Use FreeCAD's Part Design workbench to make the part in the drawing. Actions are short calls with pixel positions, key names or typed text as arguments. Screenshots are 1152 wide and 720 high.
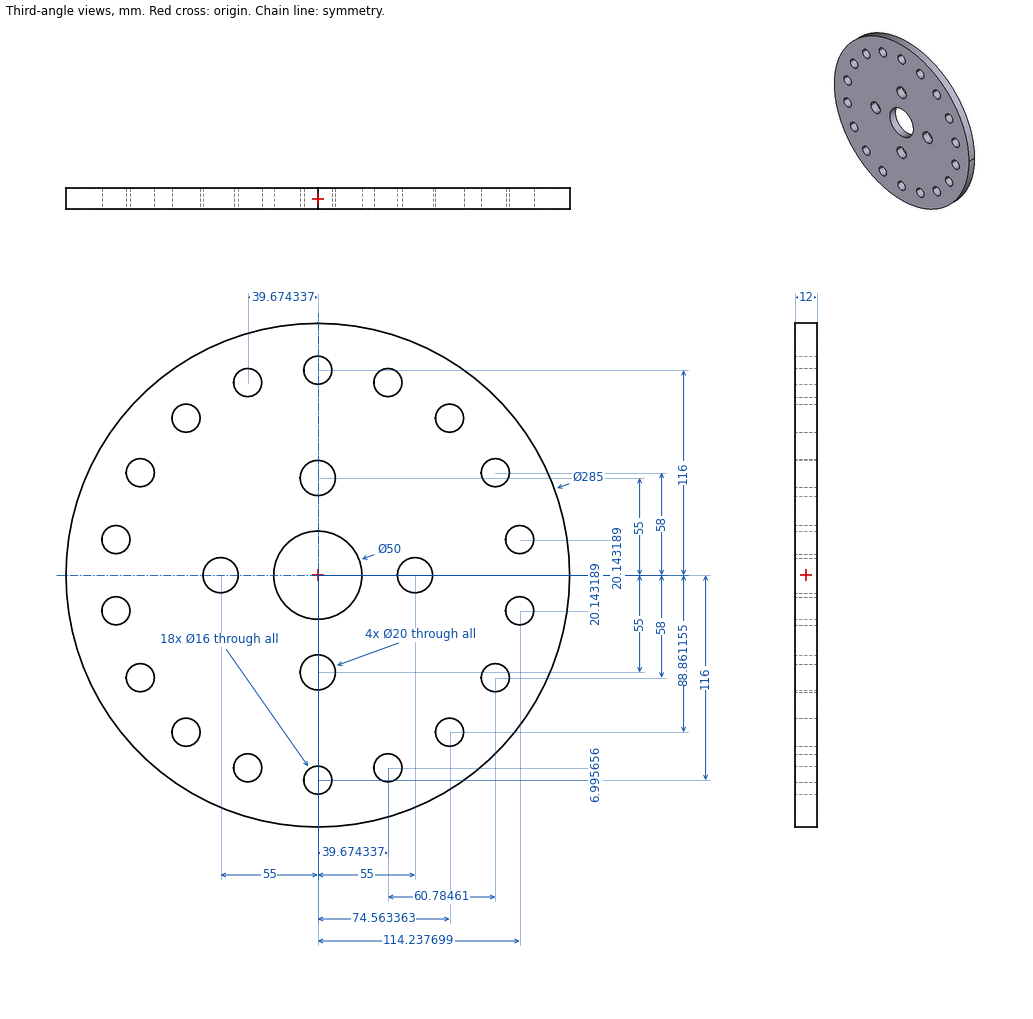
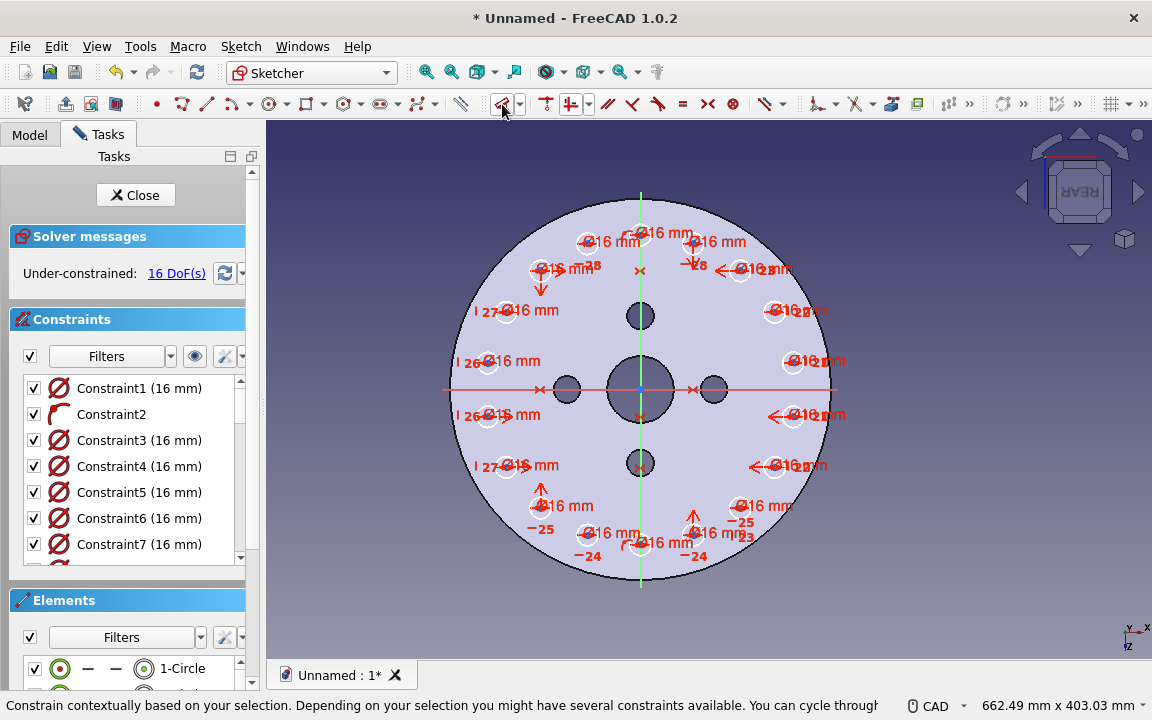
click(775, 312)
click(809, 333)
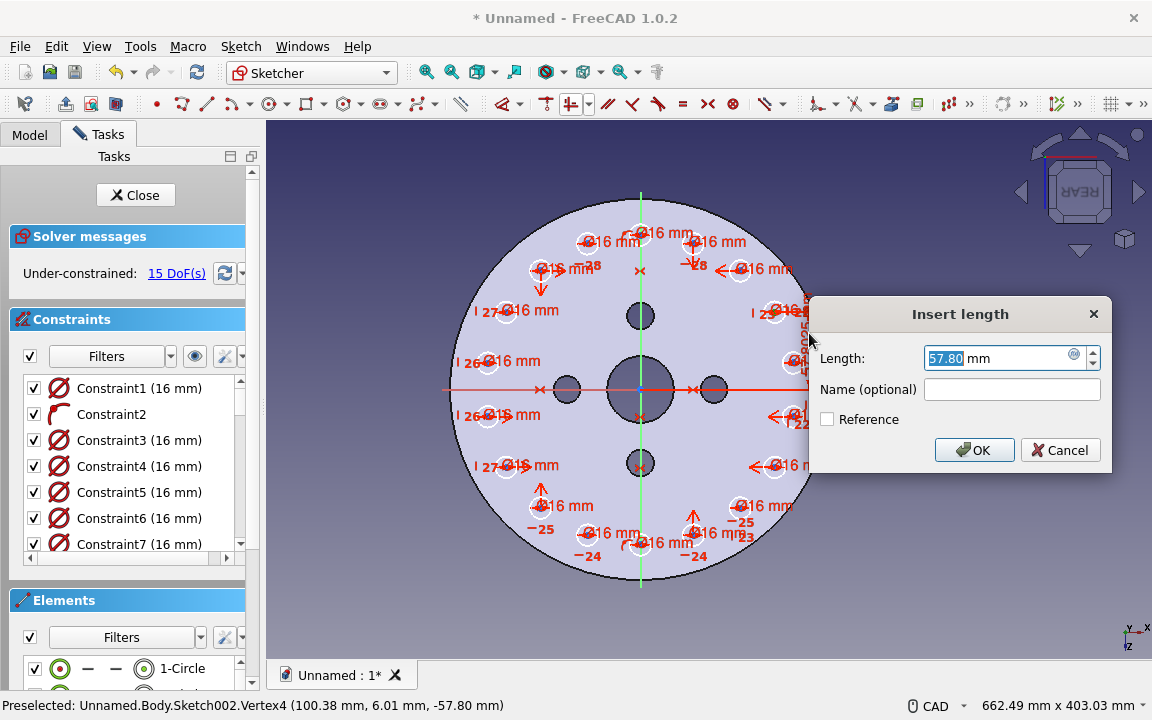
text(58)
key(Return)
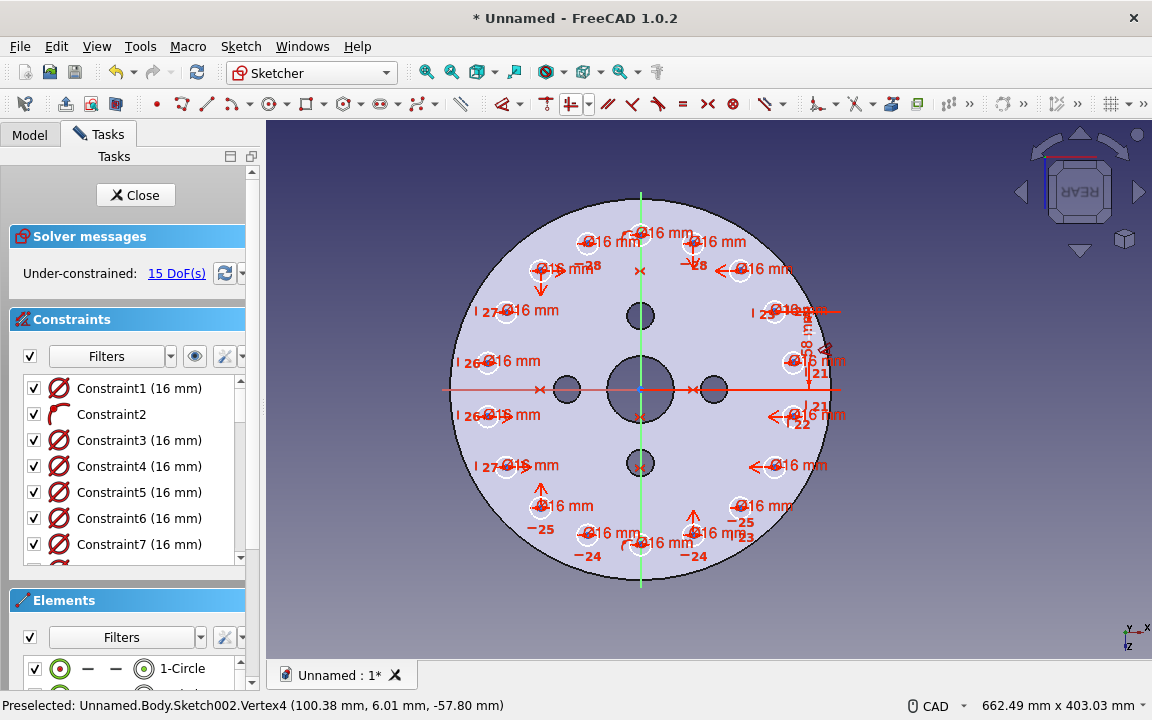
click(775, 467)
click(809, 446)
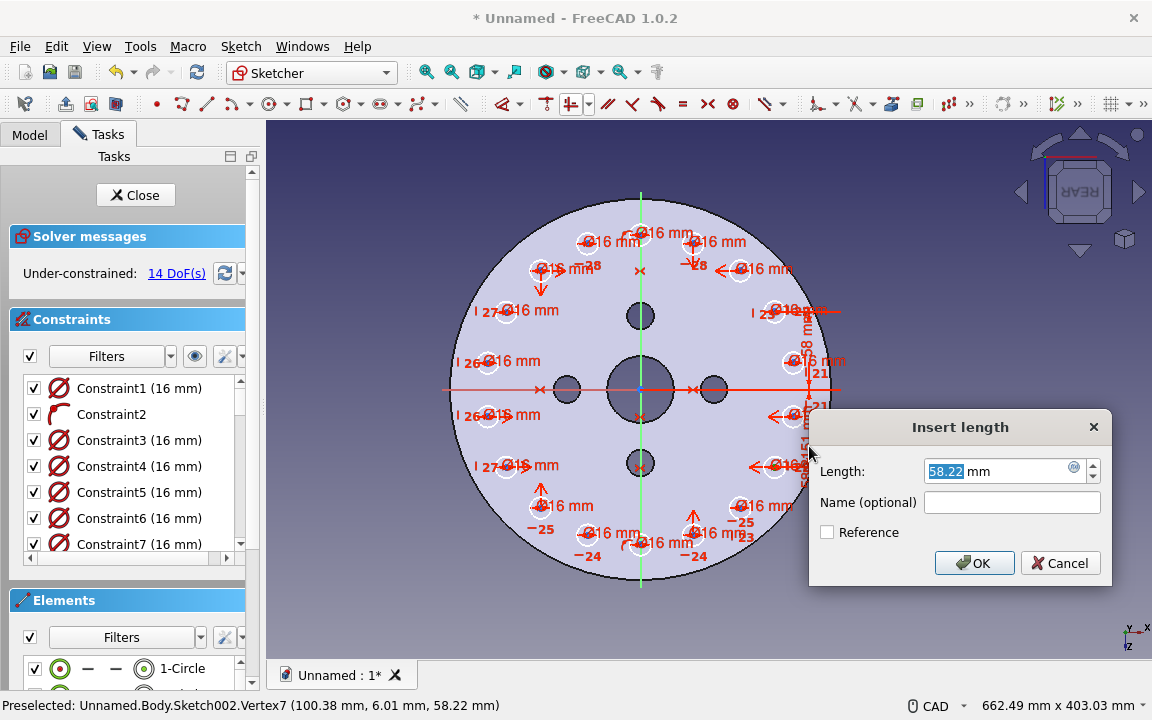
text(58)
key(Return)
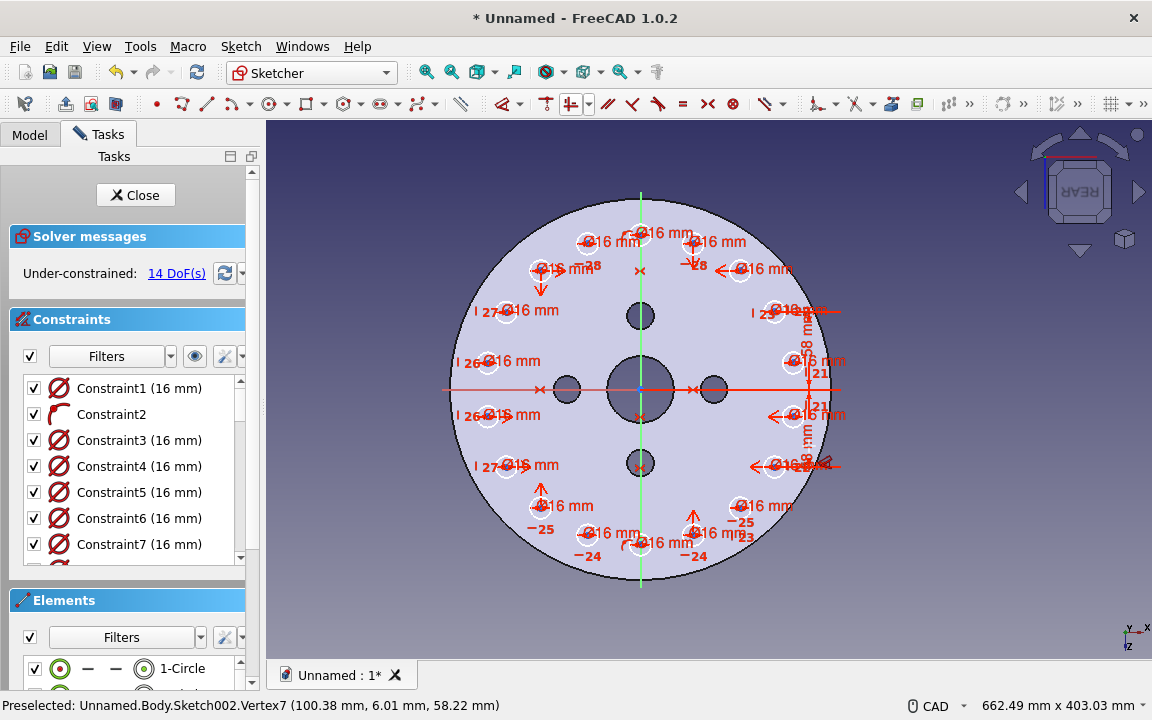
click(506, 312)
click(472, 333)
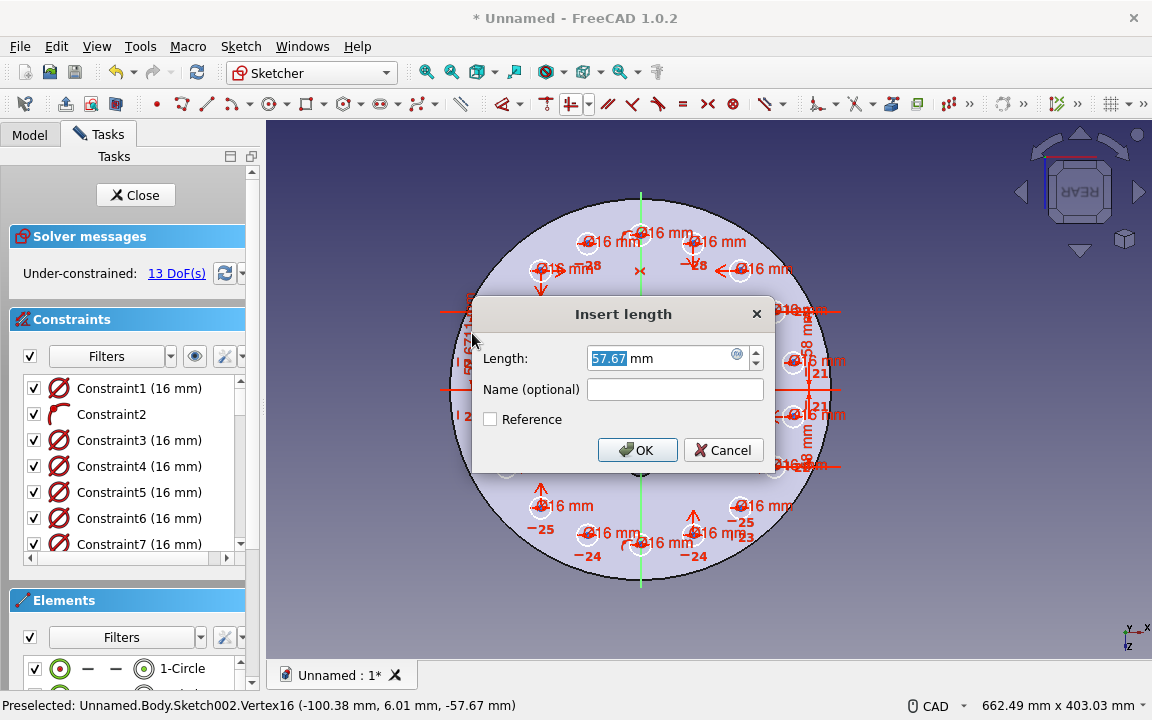
text(58)
key(Return)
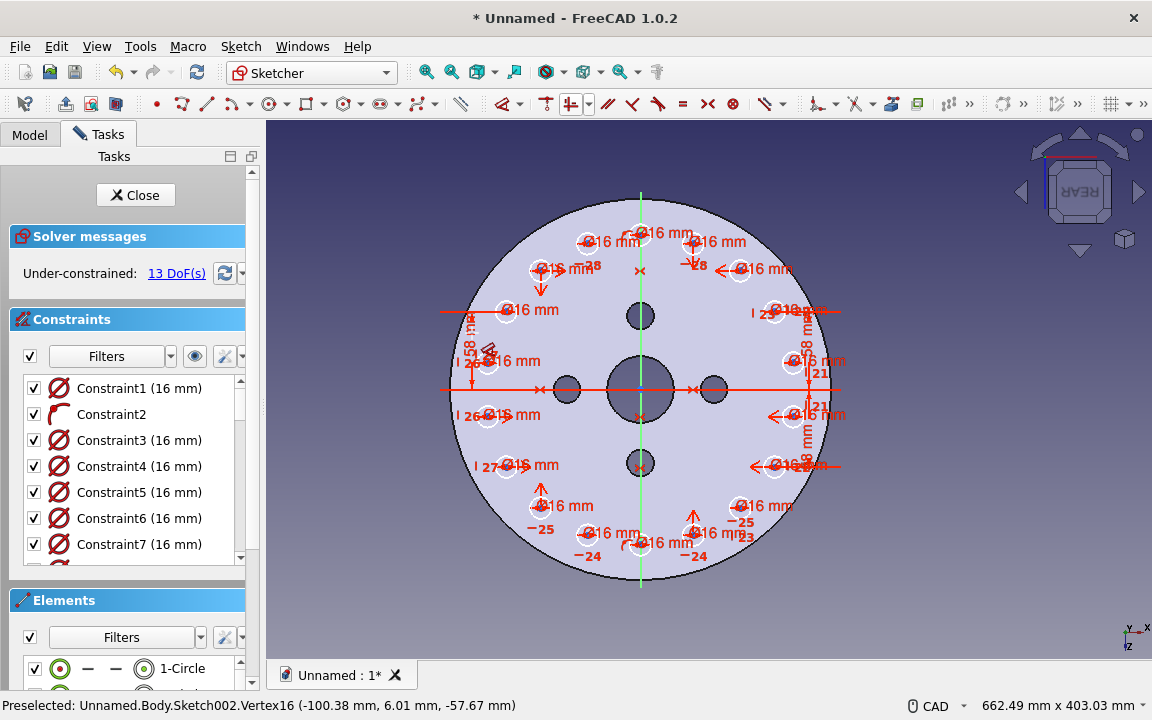
click(641, 235)
click(675, 312)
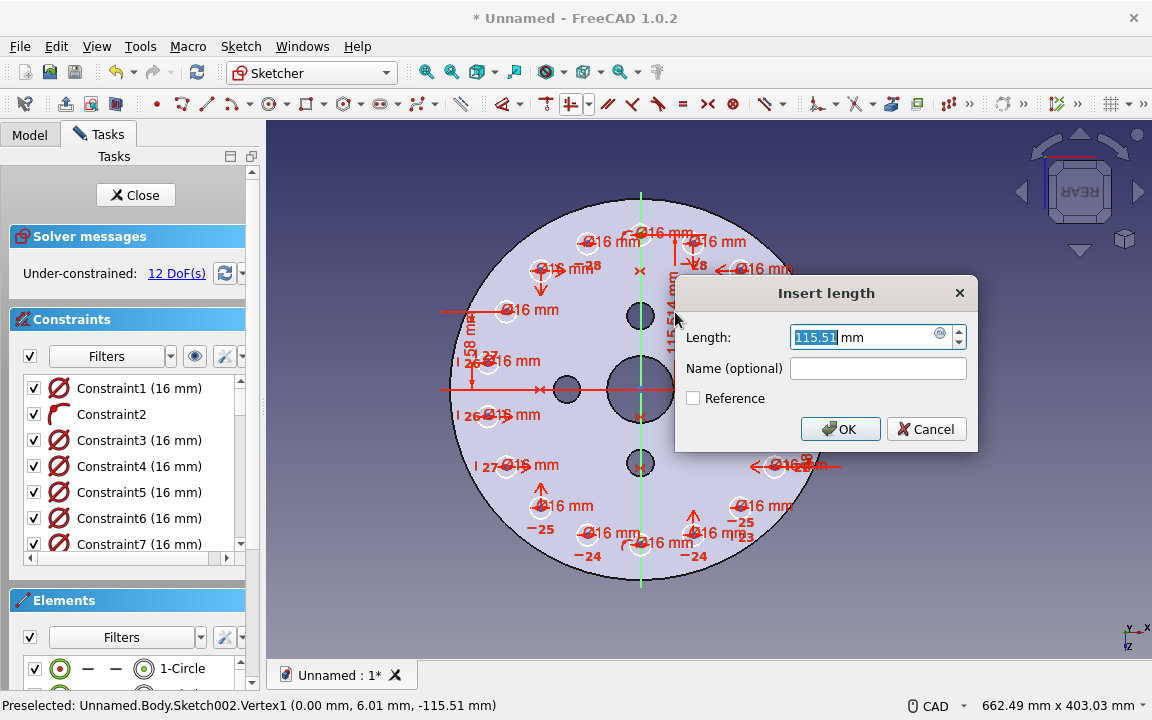
text(116)
key(Return)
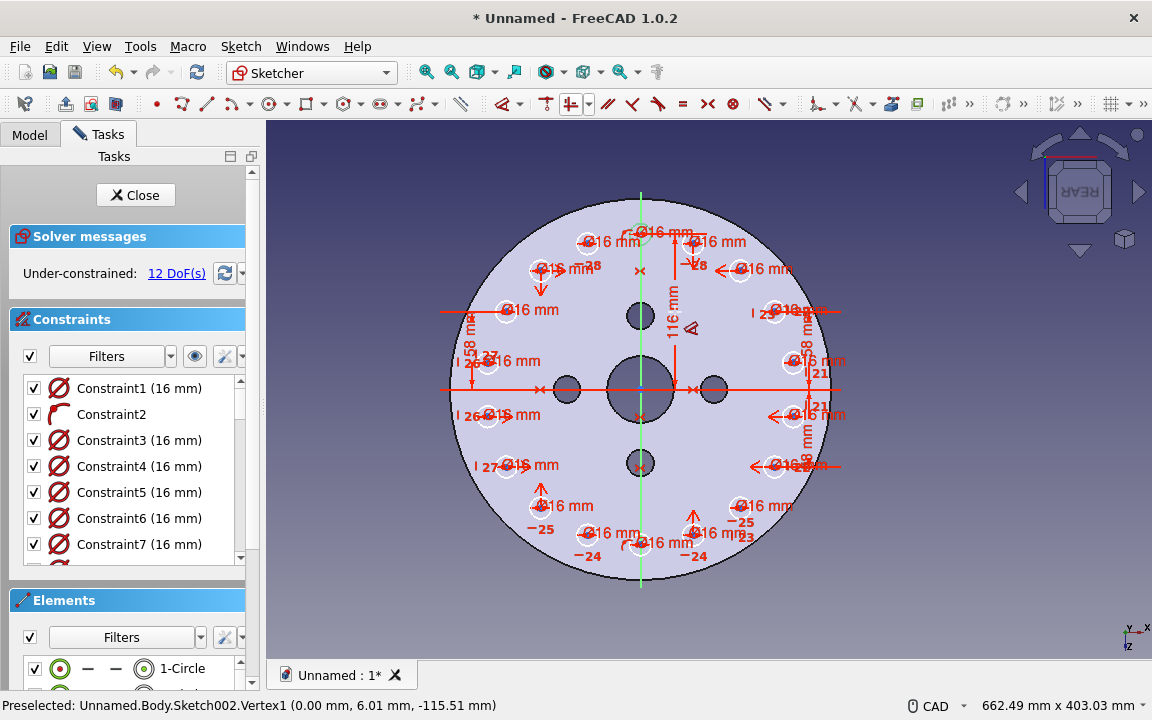
click(641, 545)
click(675, 467)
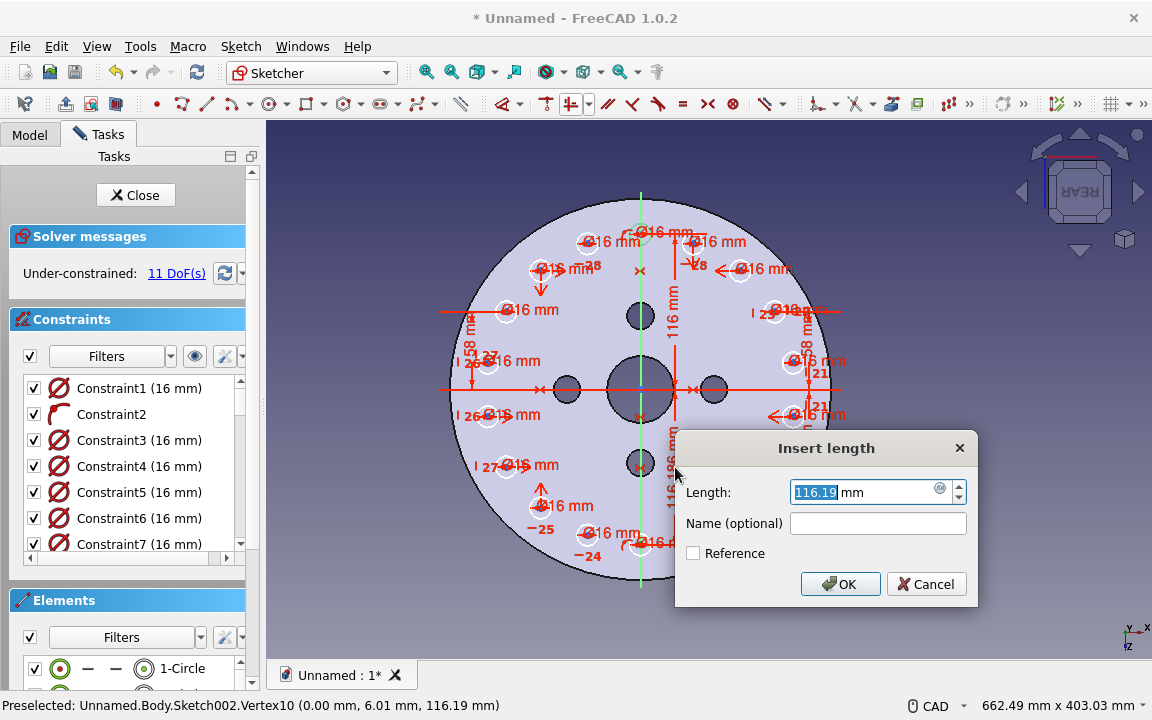
text(116)
key(Return)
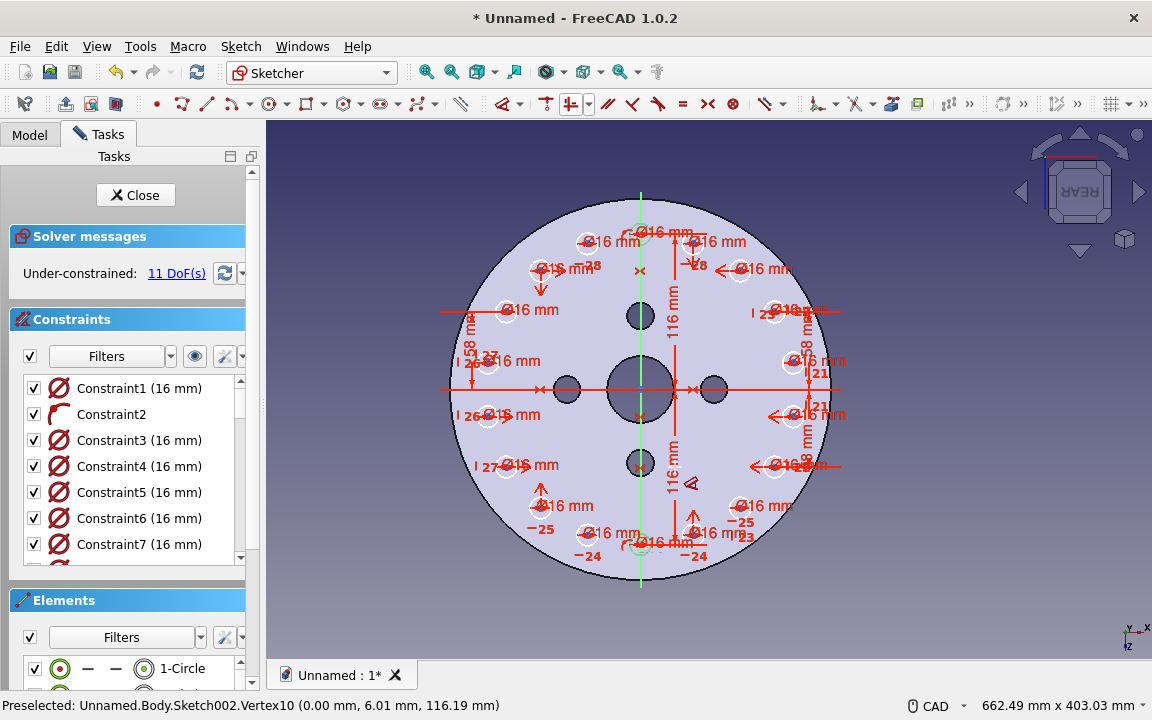
click(693, 244)
click(667, 210)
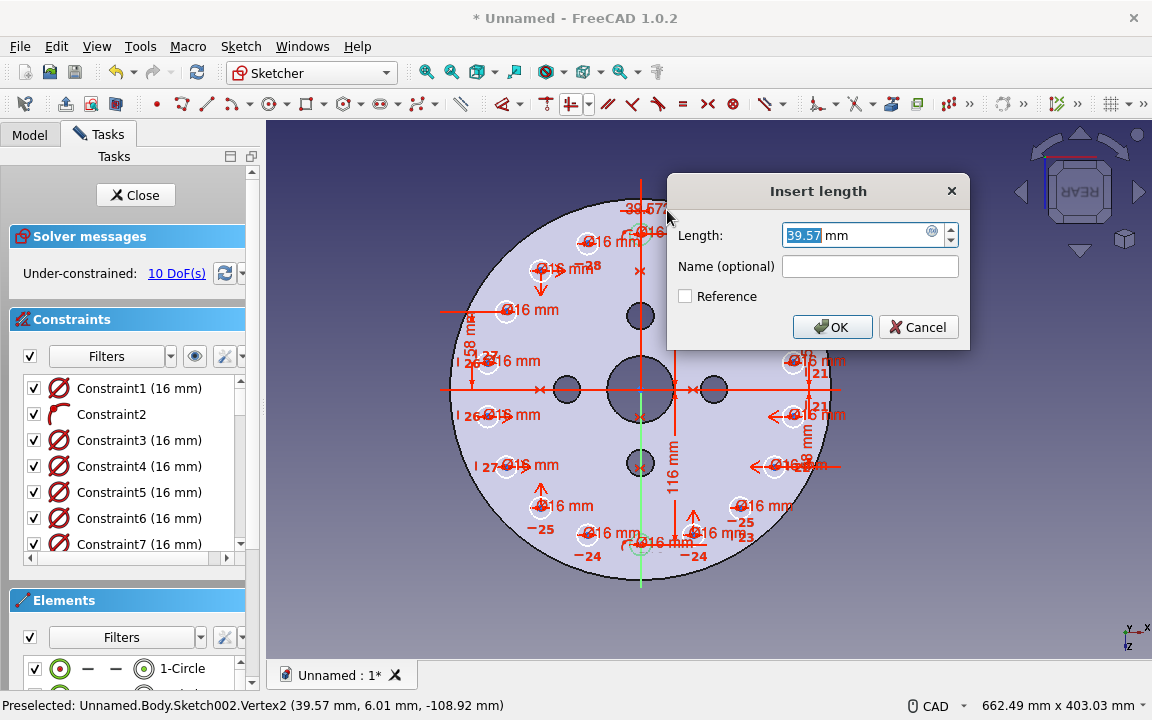
text(39.674337)
key(Return)